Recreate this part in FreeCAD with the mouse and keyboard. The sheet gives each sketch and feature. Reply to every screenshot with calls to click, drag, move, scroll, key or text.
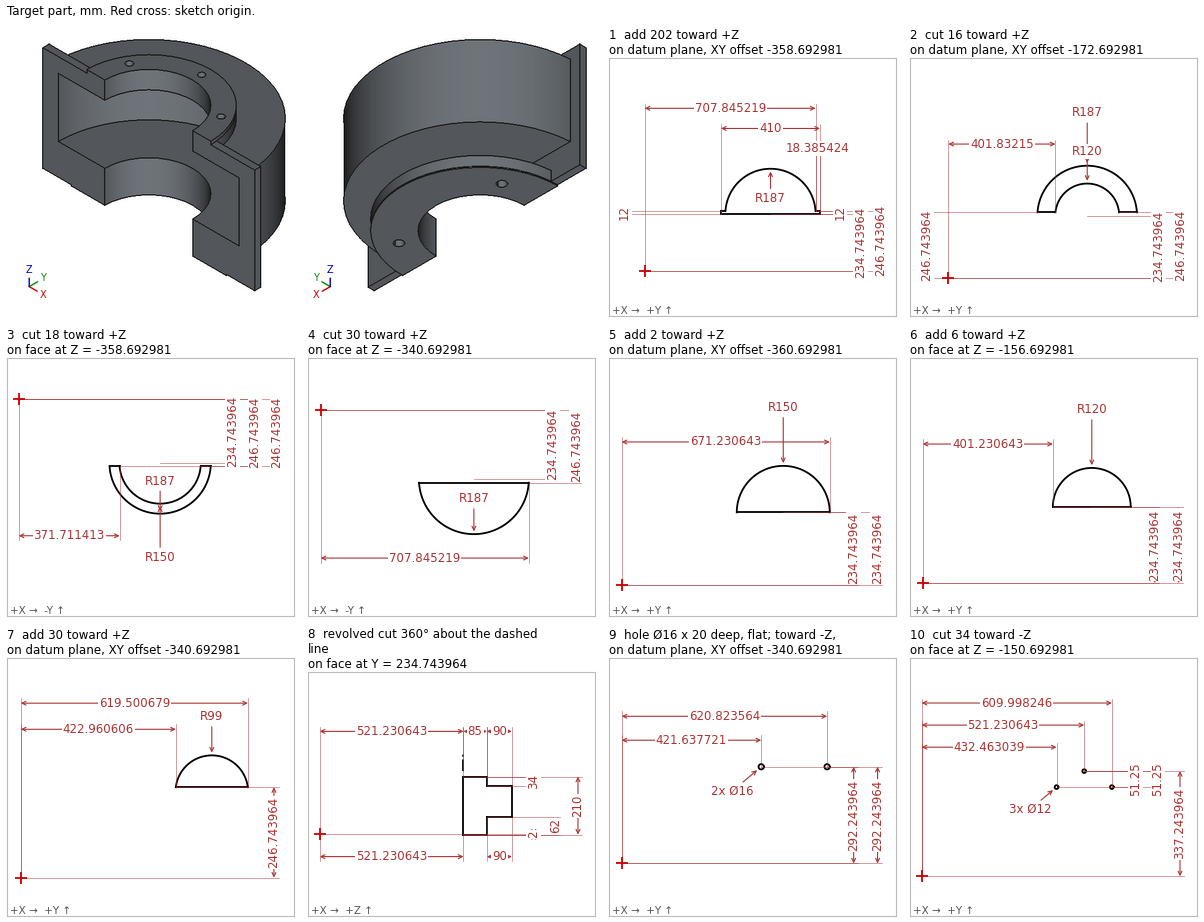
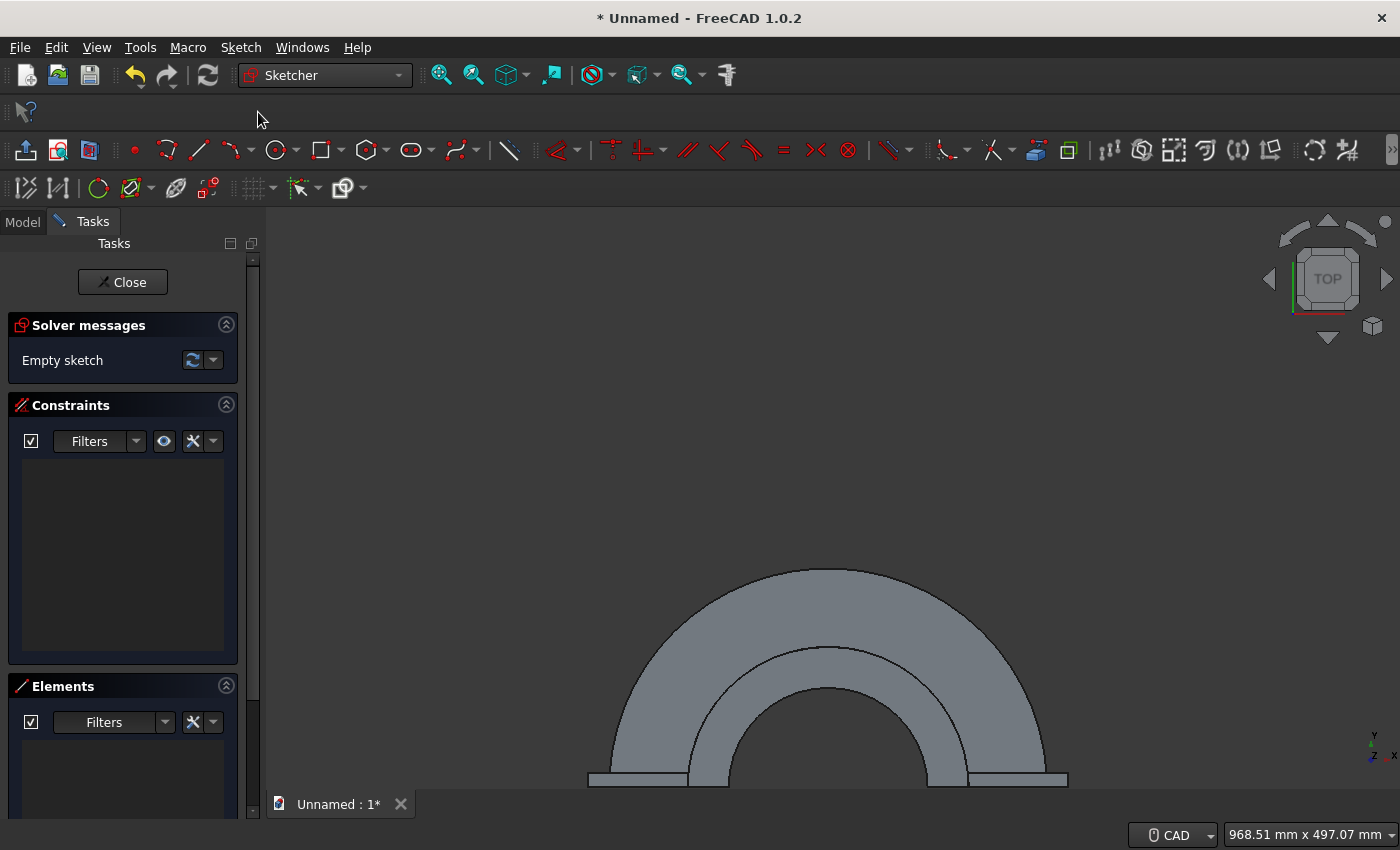
scroll(865, 761, up, 5)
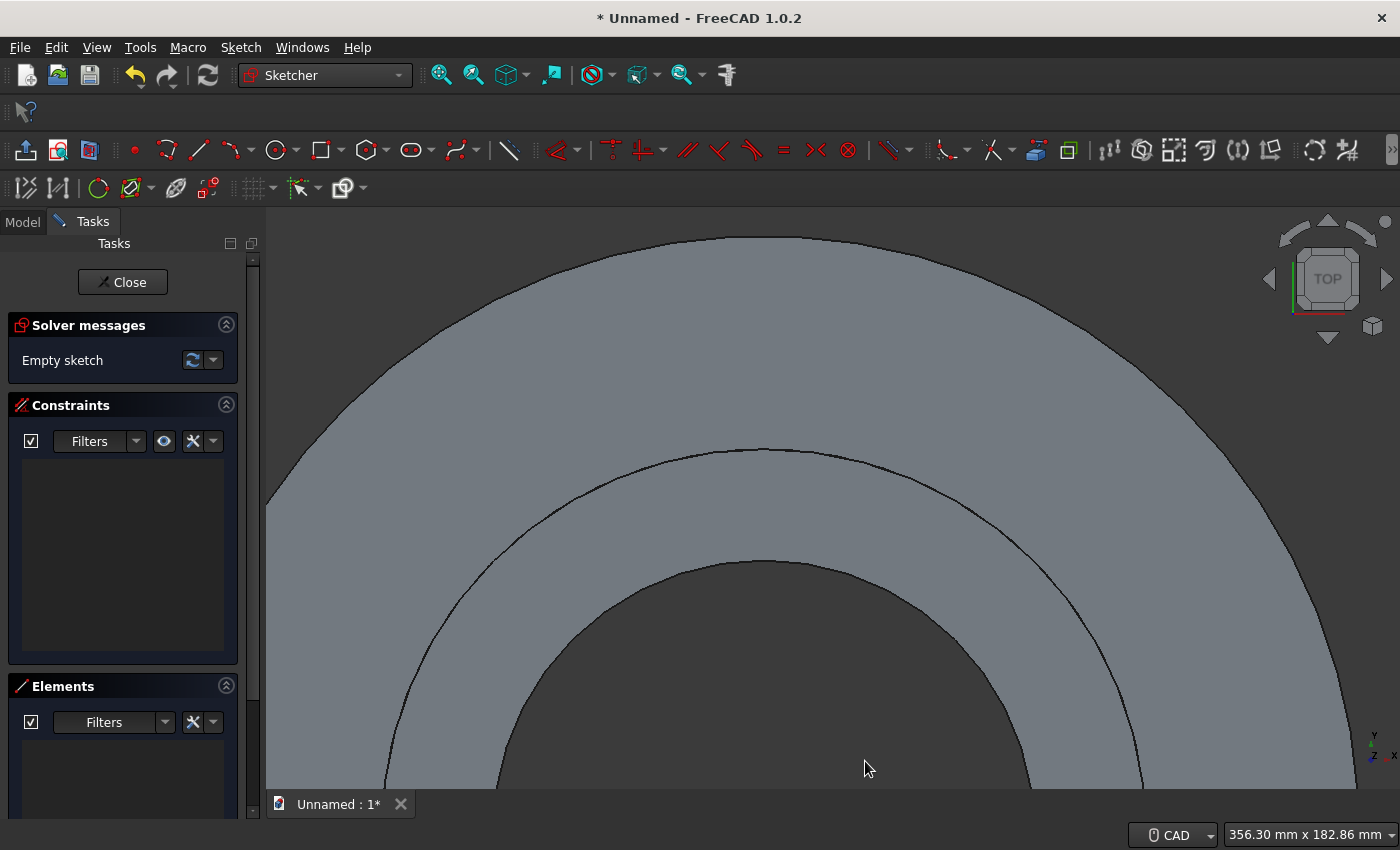
key(g)
key(c)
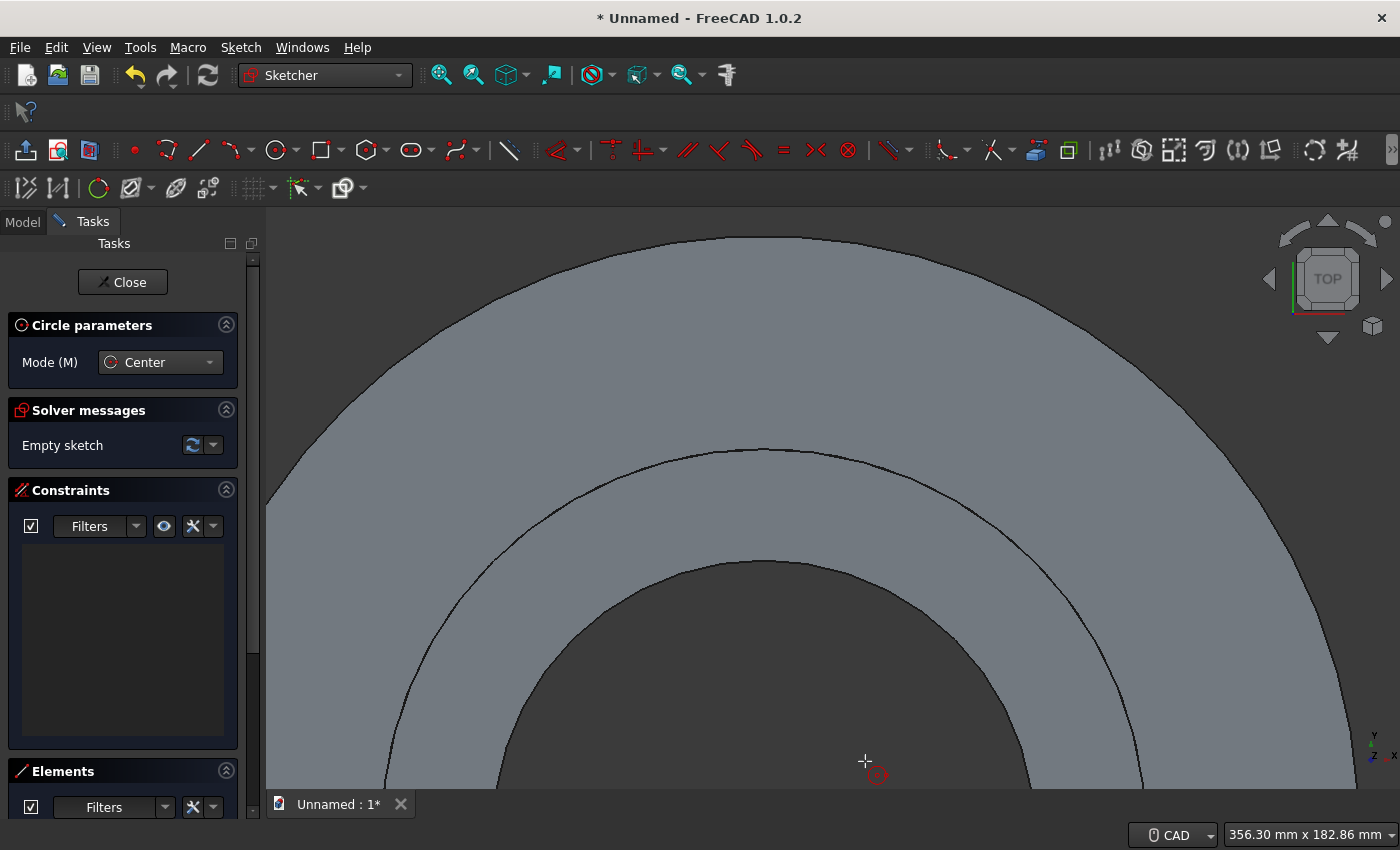
click(764, 505)
move(777, 491)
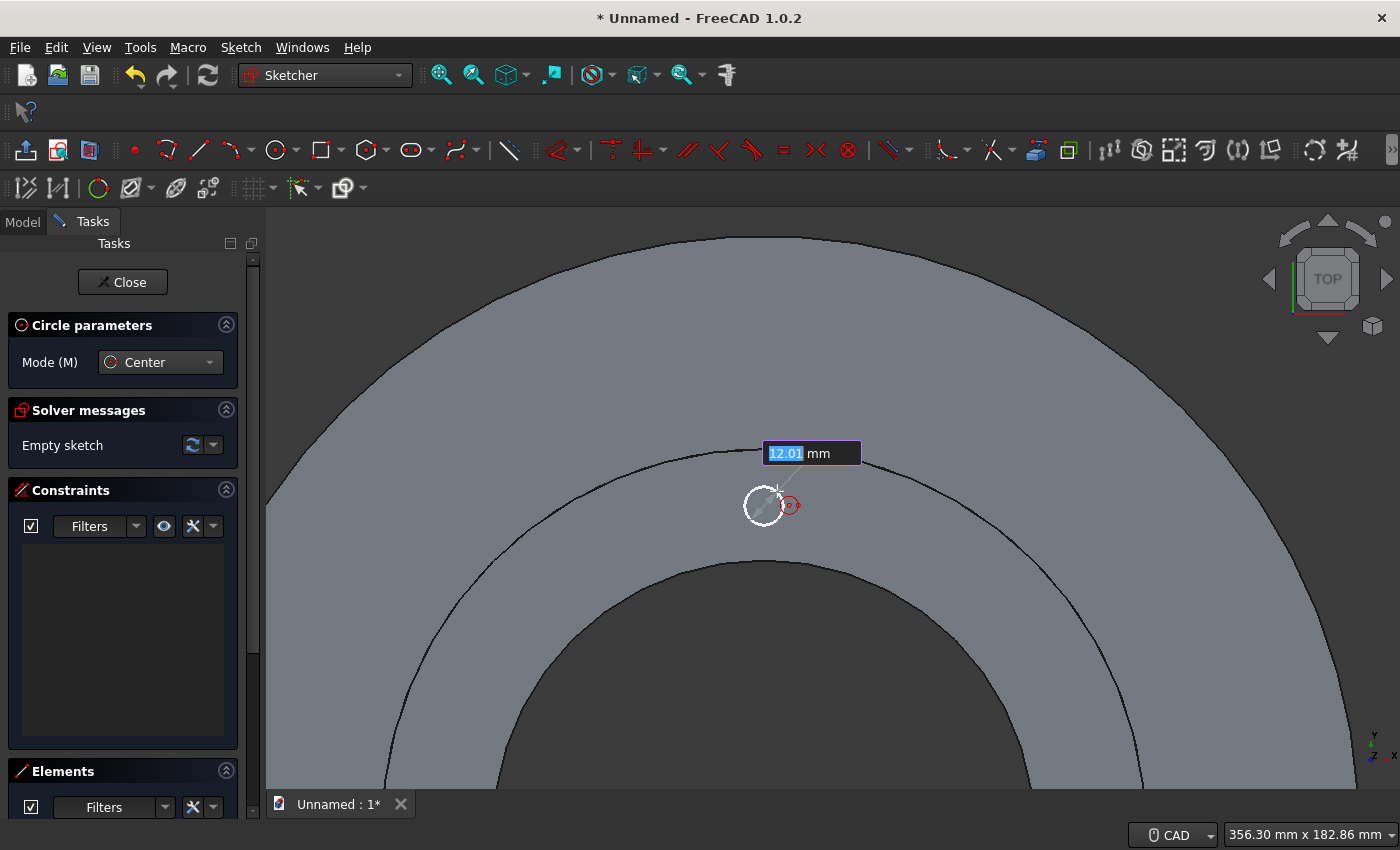
text(12)
key(Return)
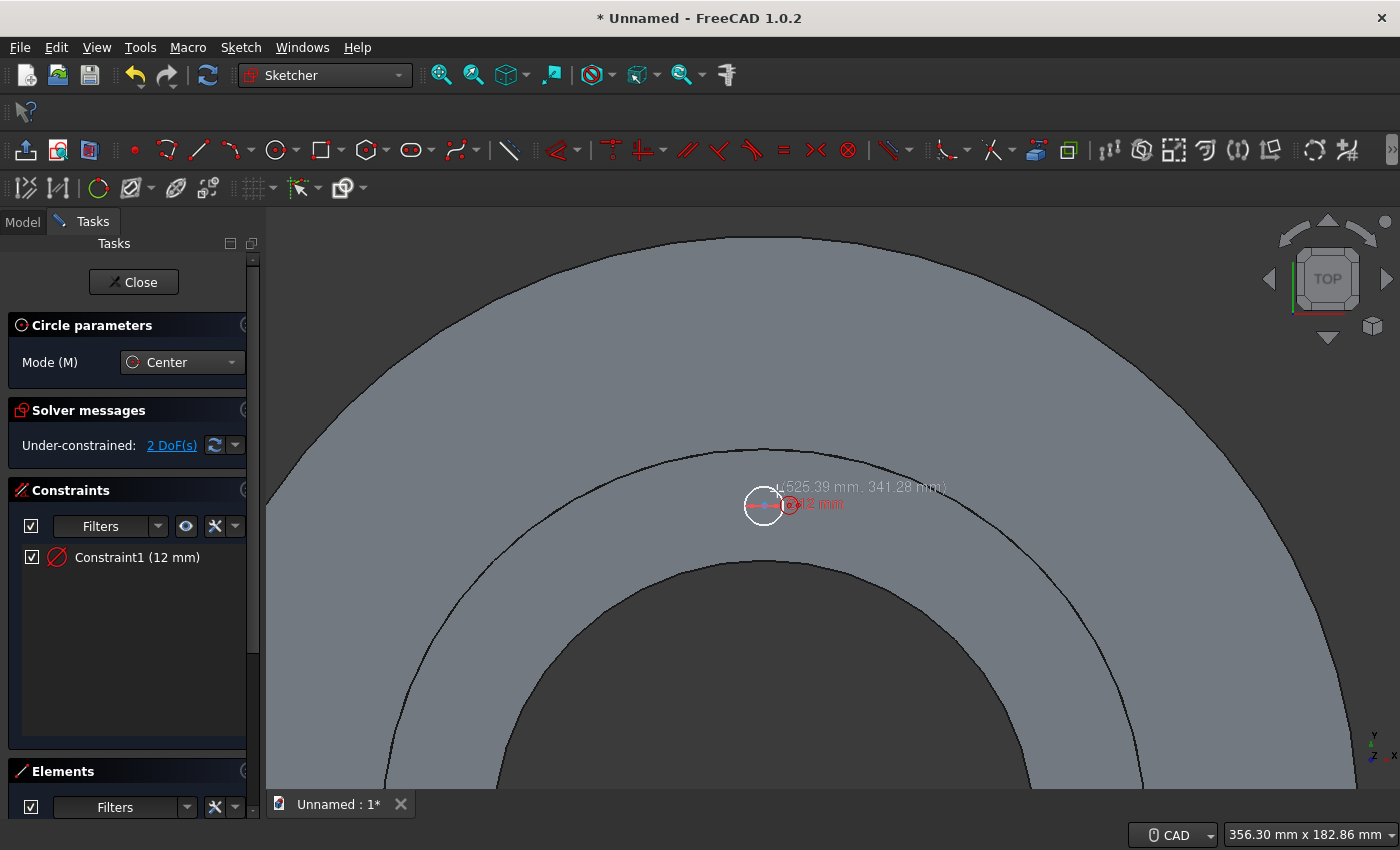
click(481, 668)
move(495, 654)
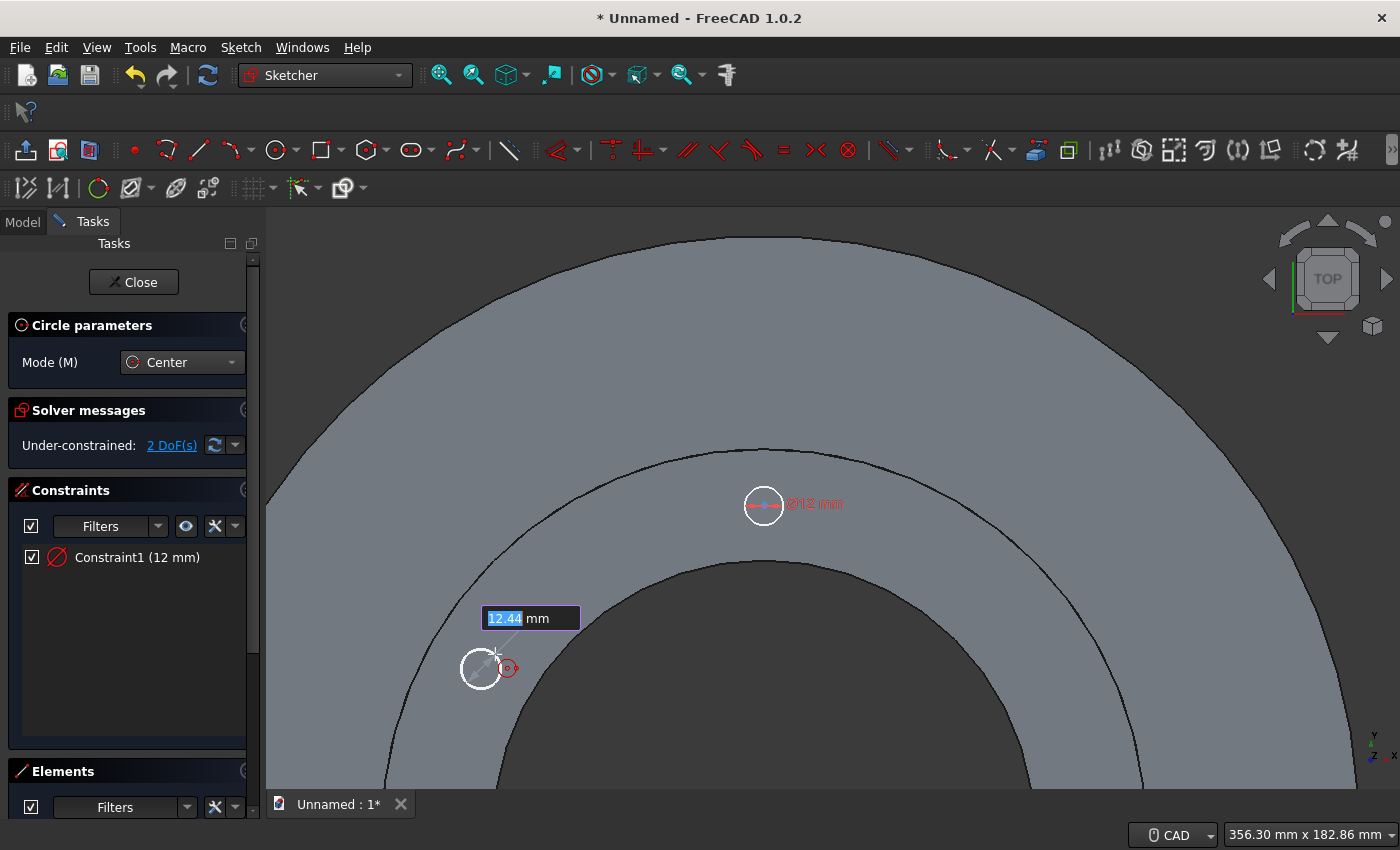
text(12)
key(Return)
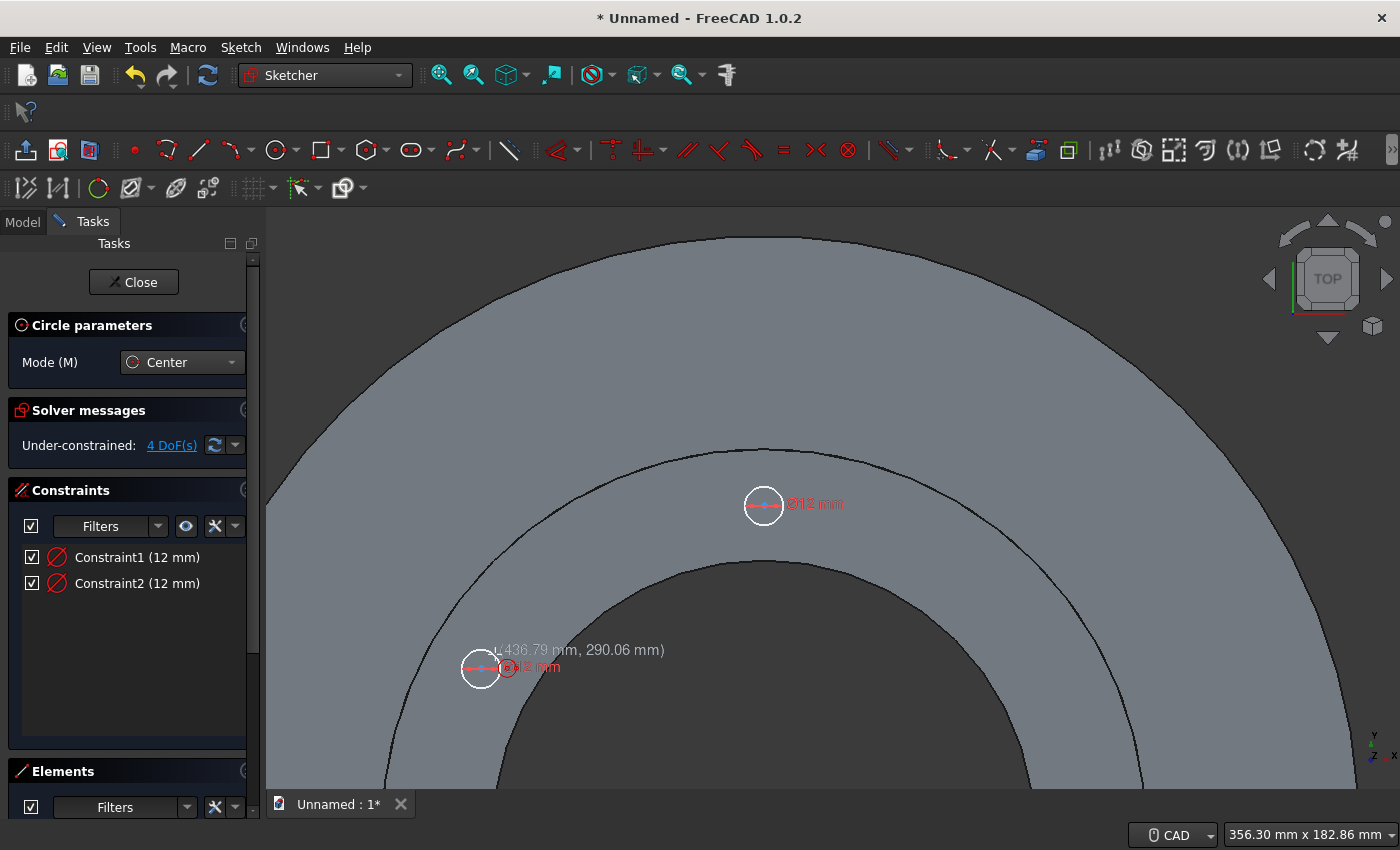
click(1046, 668)
move(1060, 654)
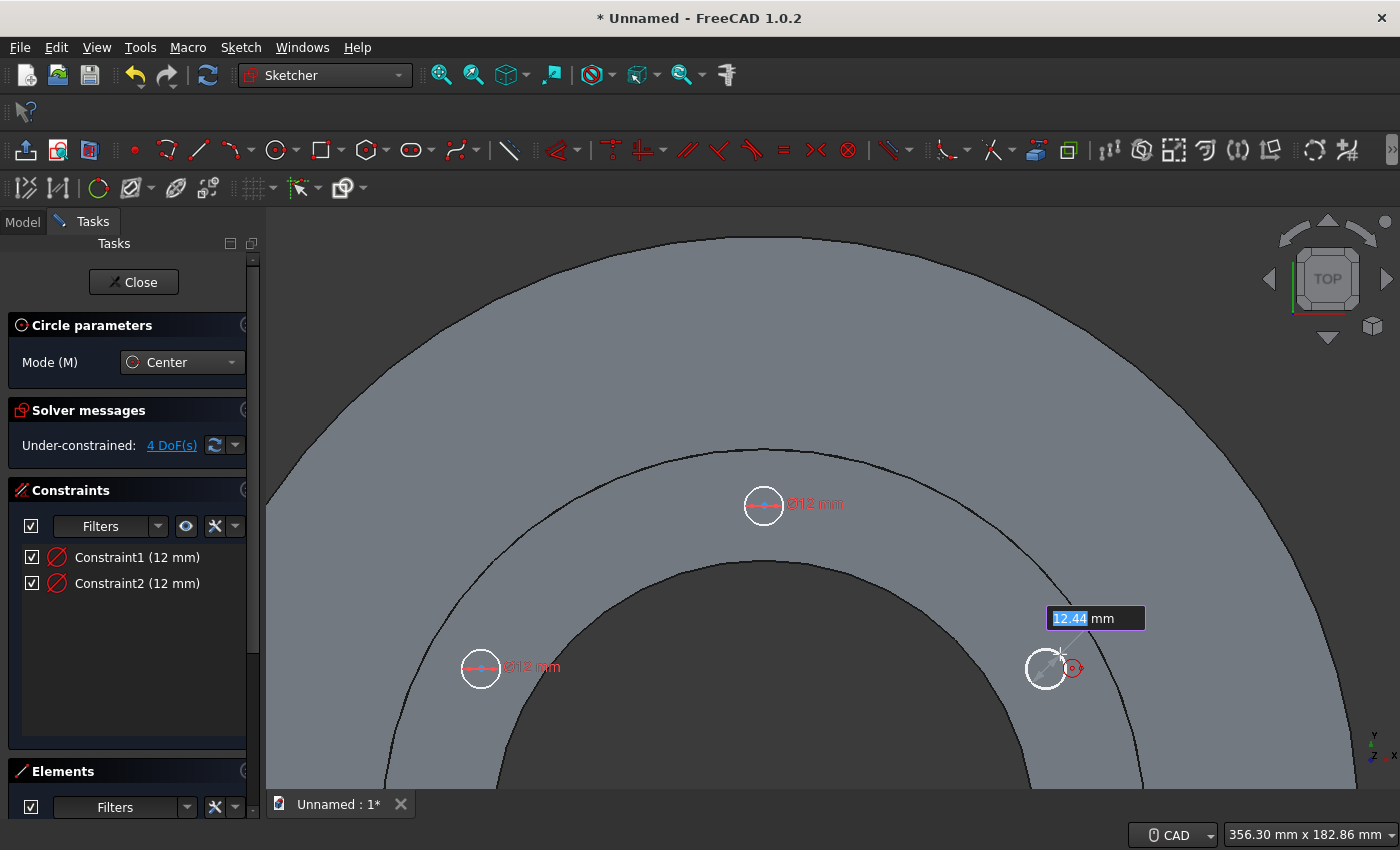
text(12)
key(Return)
key(Escape)